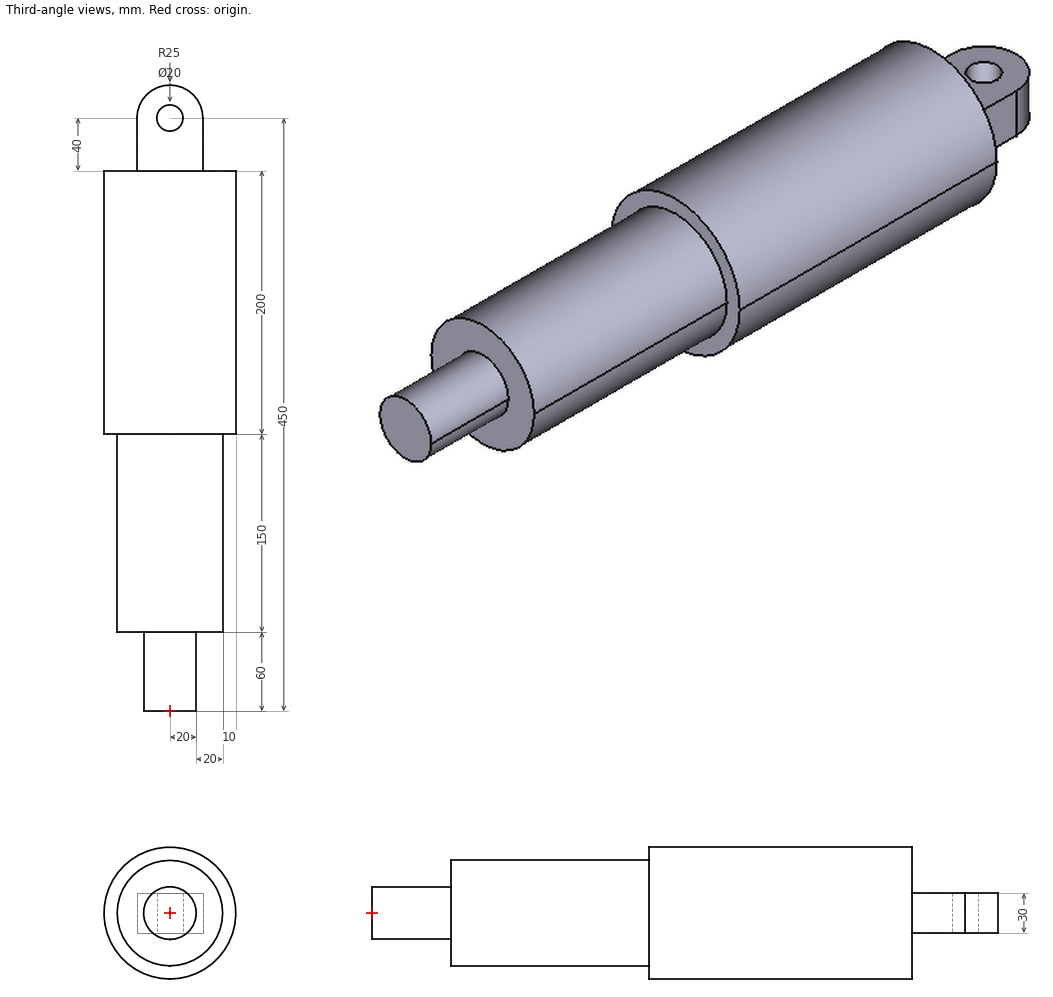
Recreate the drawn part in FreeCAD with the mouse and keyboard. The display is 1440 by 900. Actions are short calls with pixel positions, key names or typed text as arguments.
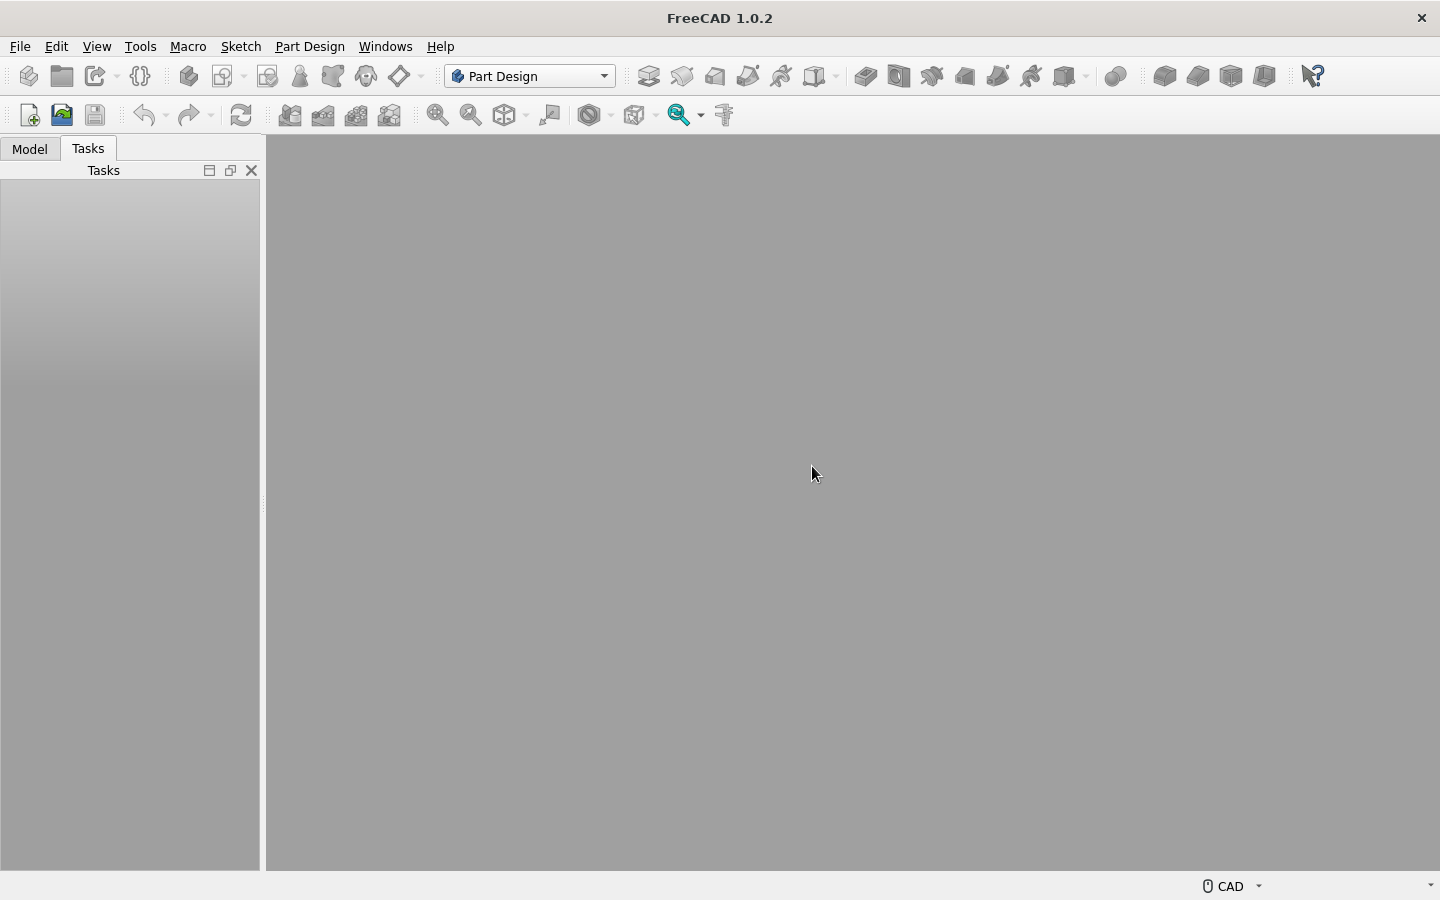
click(29, 116)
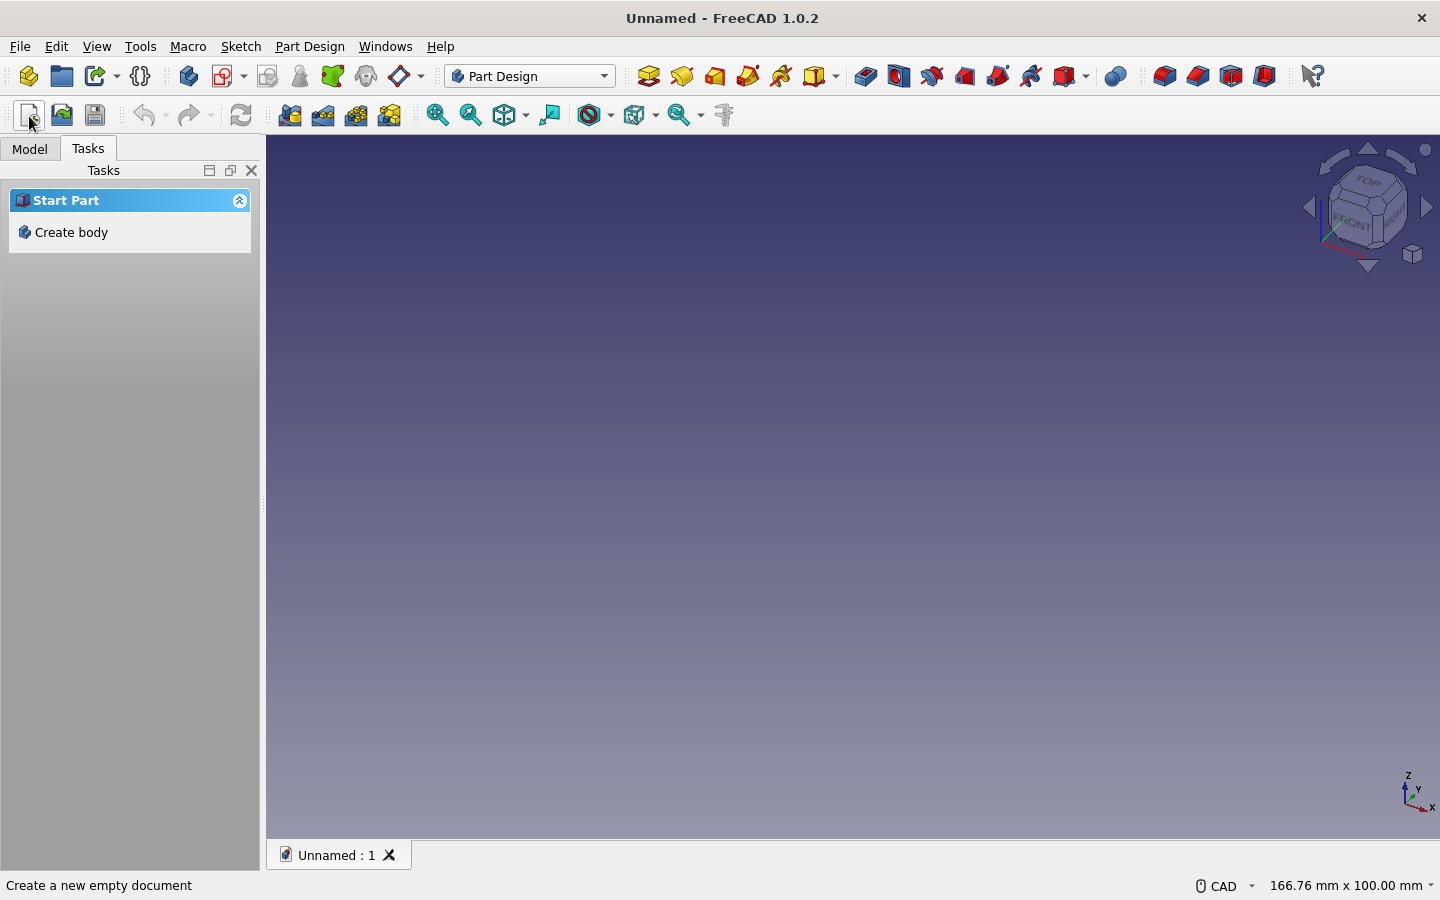
click(222, 76)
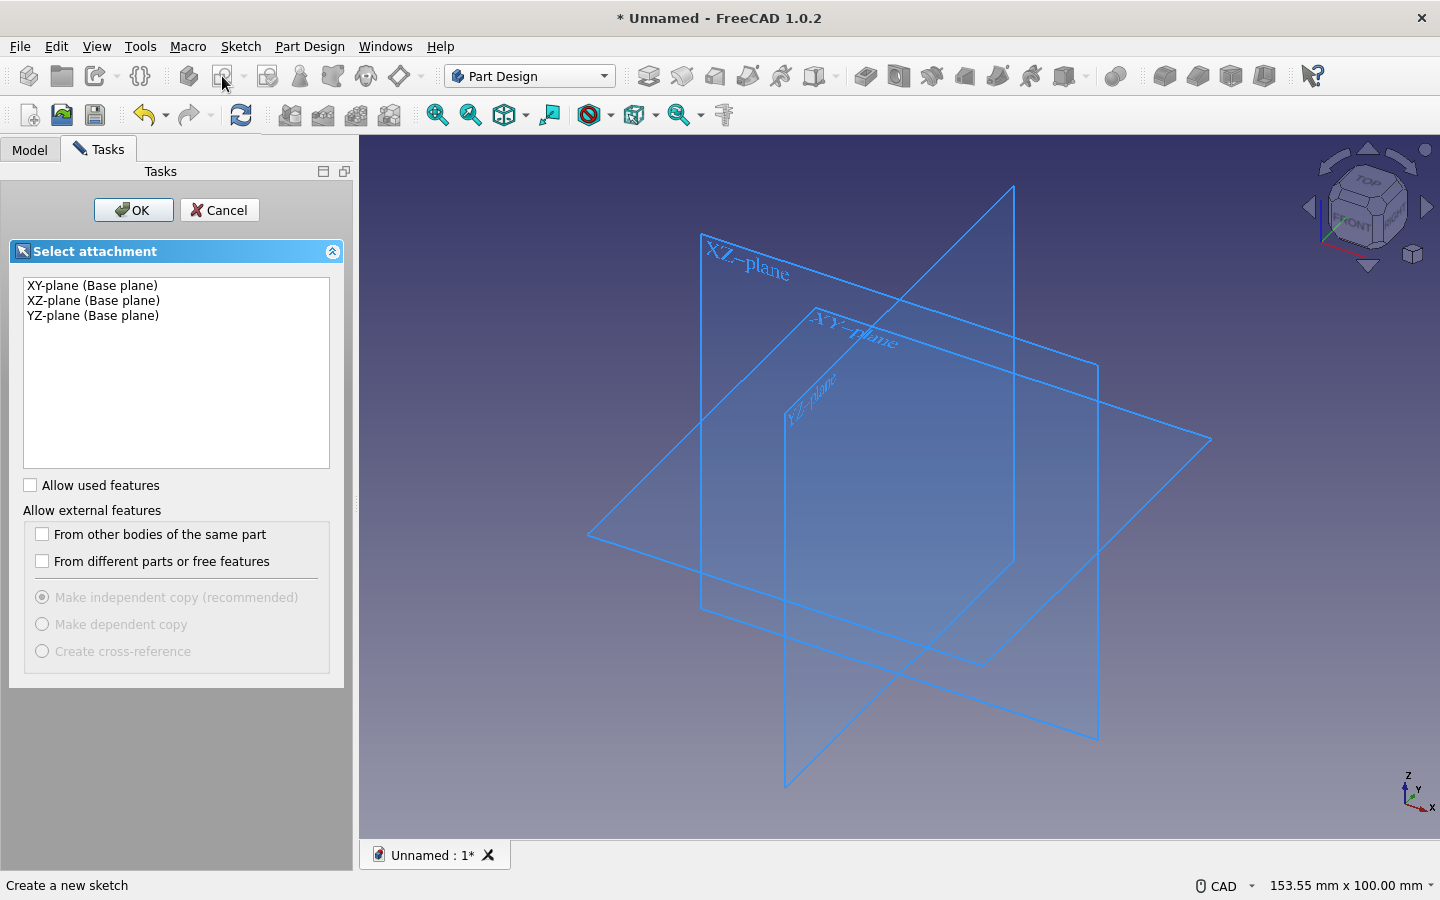
click(84, 286)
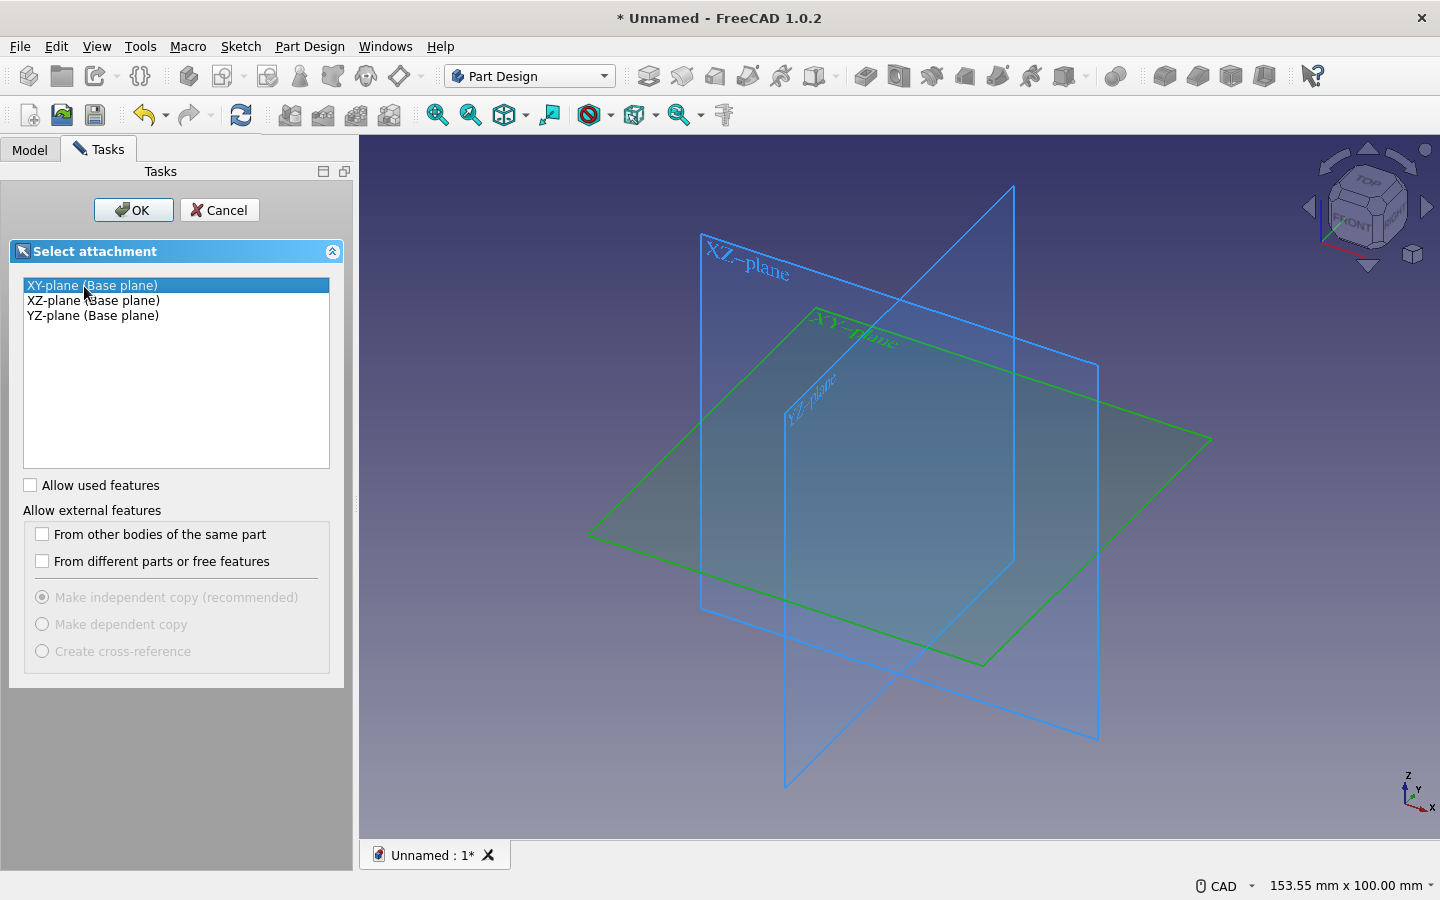
click(134, 210)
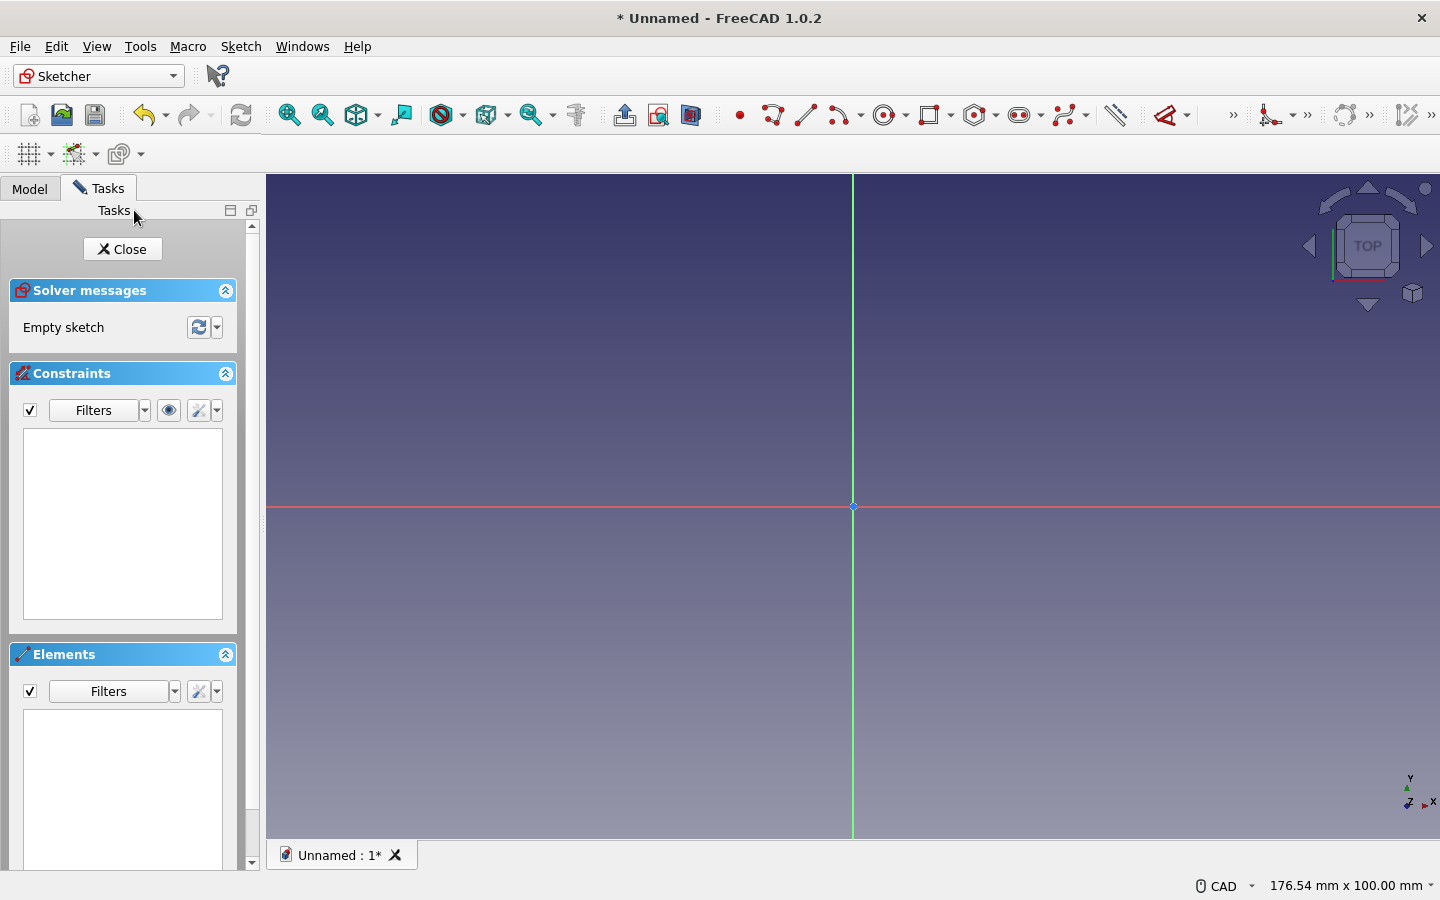
scroll(738, 776, down, 9)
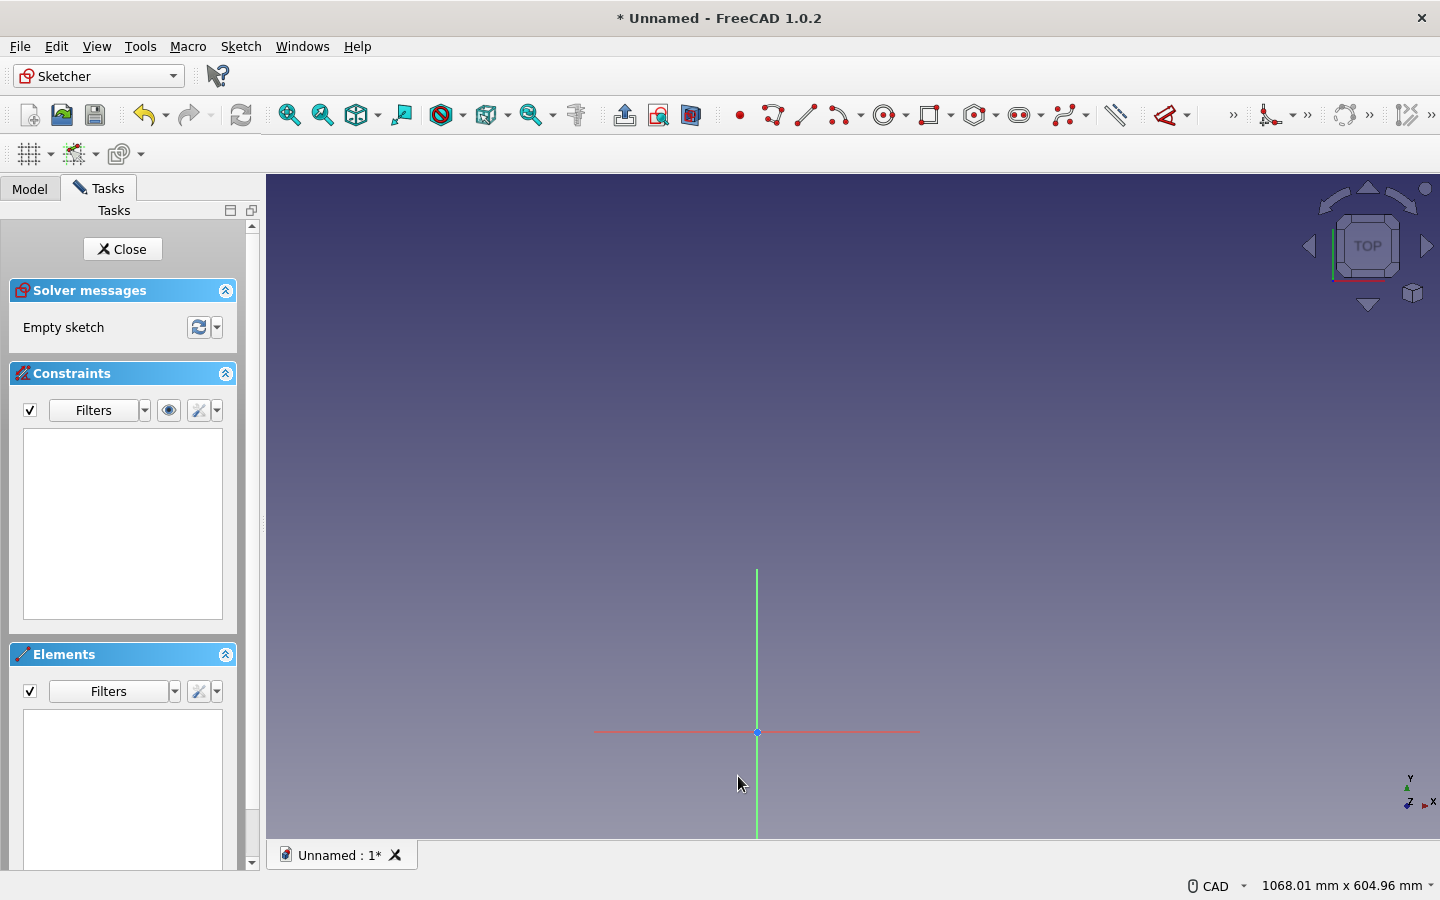
click(773, 116)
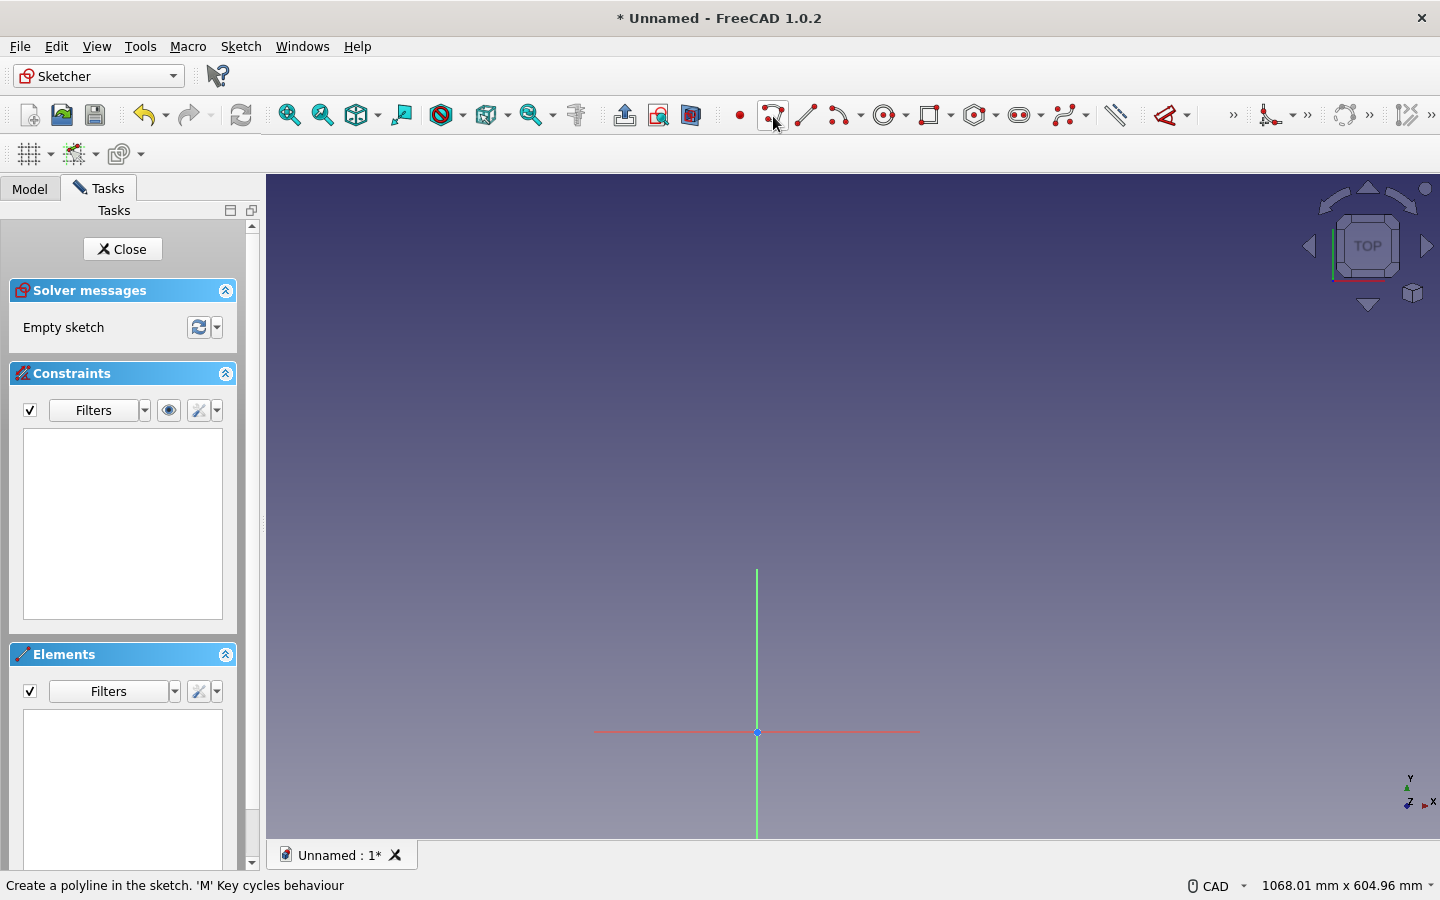
click(757, 732)
click(779, 723)
click(779, 666)
click(801, 666)
click(801, 501)